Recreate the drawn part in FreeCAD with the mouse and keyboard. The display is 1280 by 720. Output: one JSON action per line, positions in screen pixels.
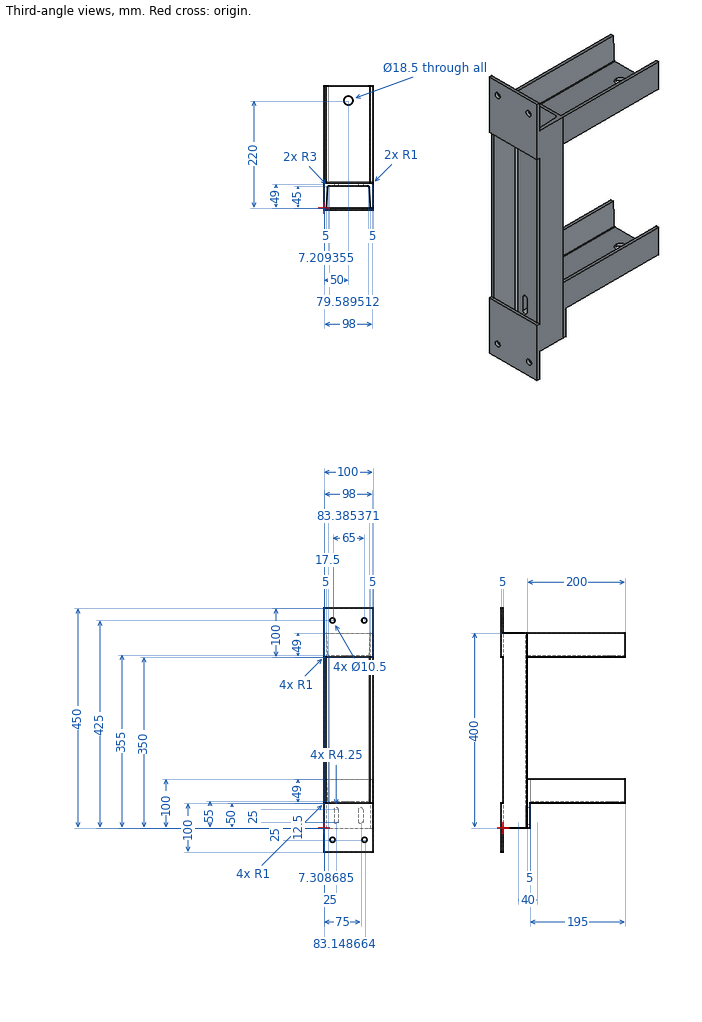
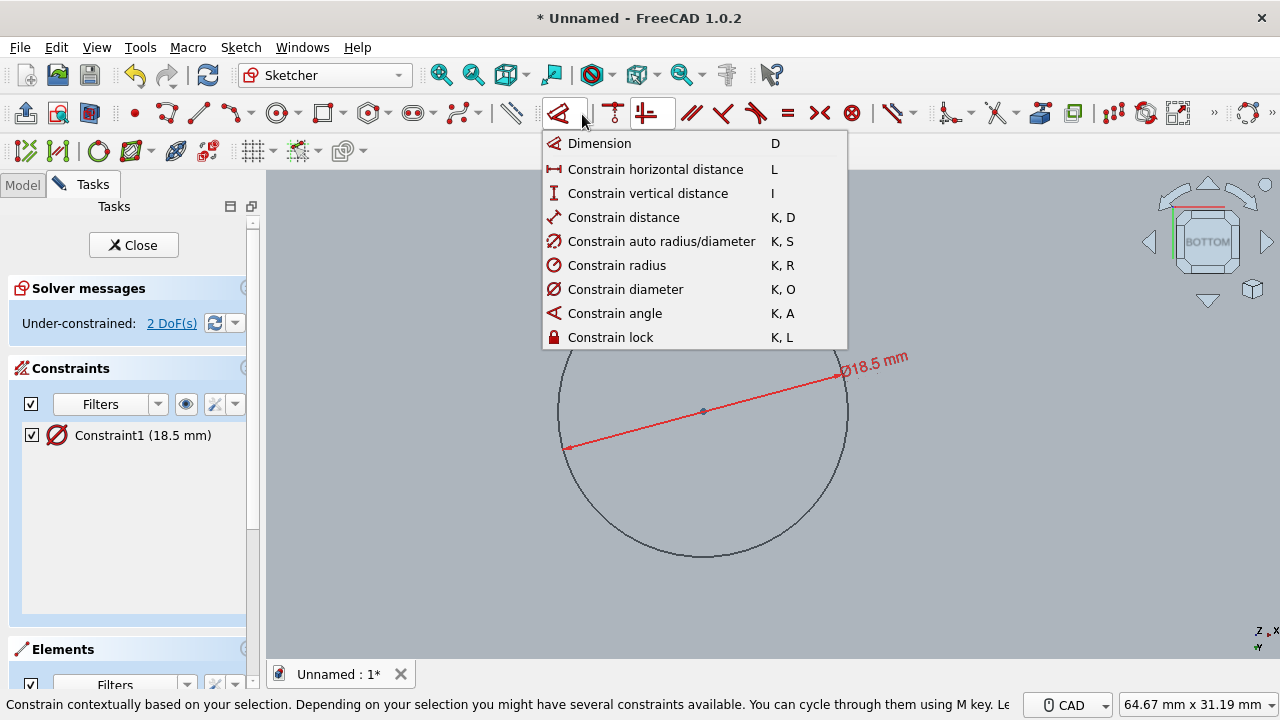
{"action": "left_click", "coordinate": [695, 169]}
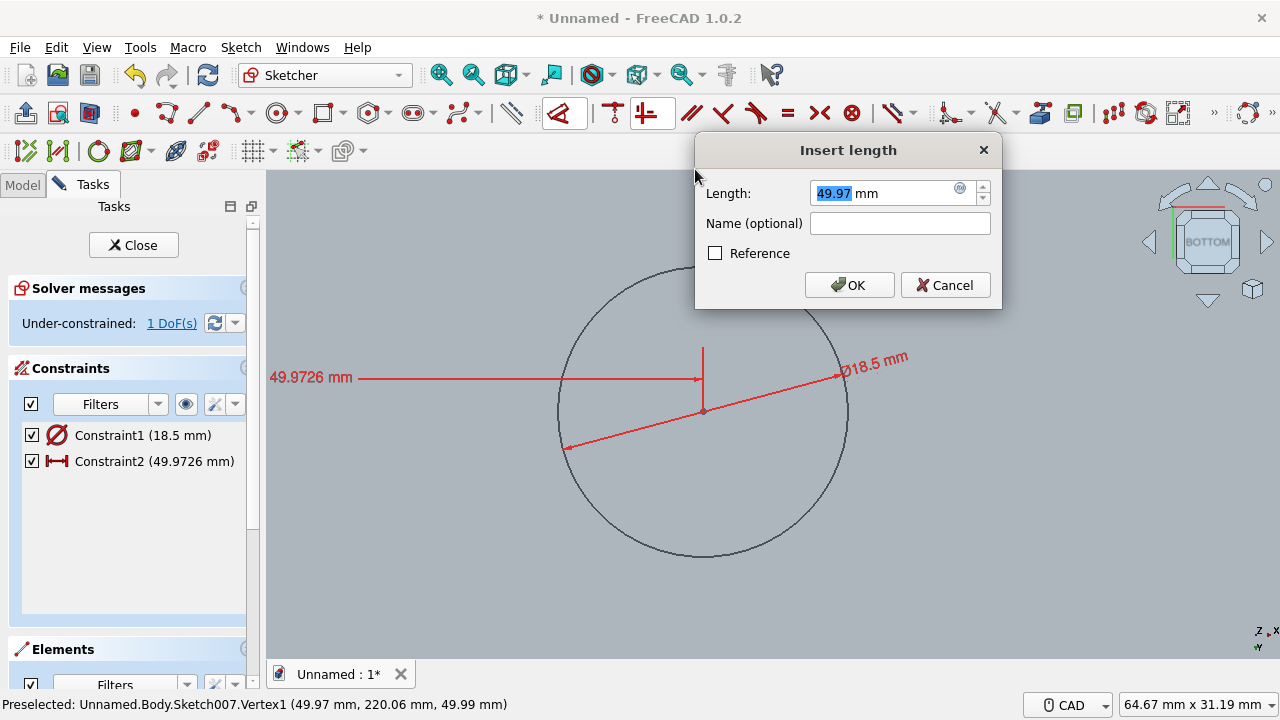
{"action": "type", "text": "50"}
{"action": "key", "text": "Return"}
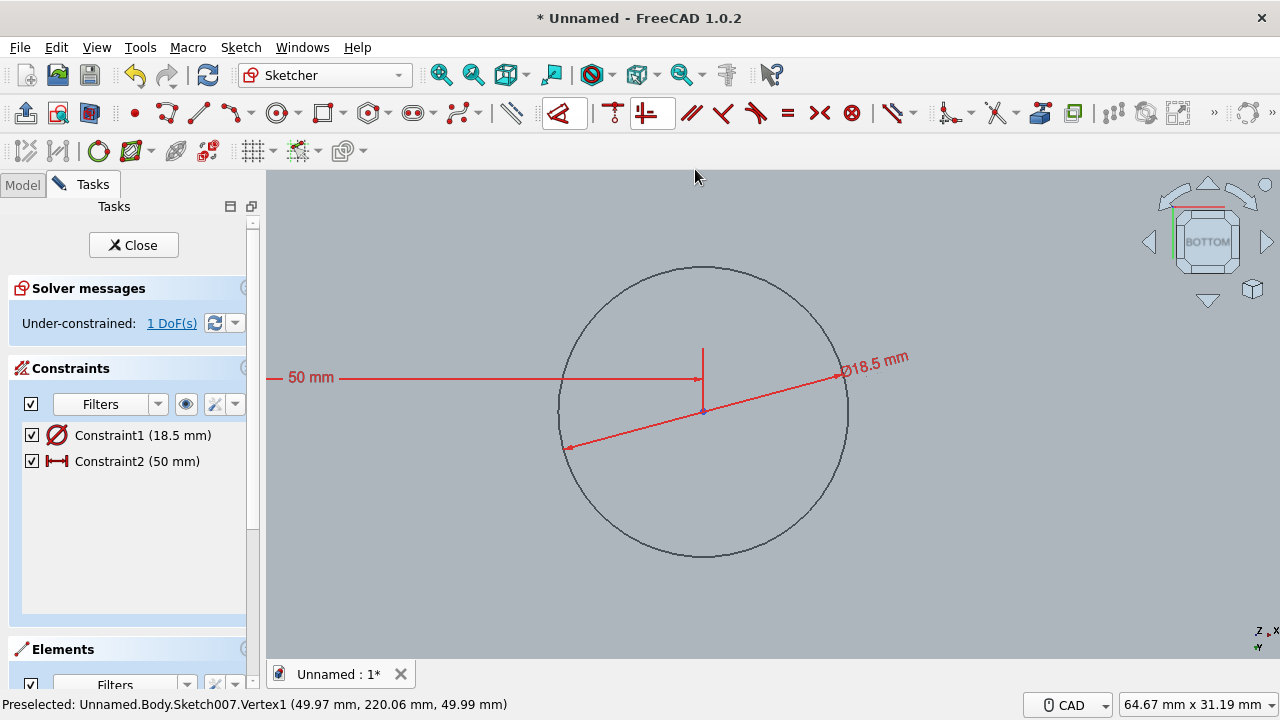
{"action": "left_click", "coordinate": [703, 412]}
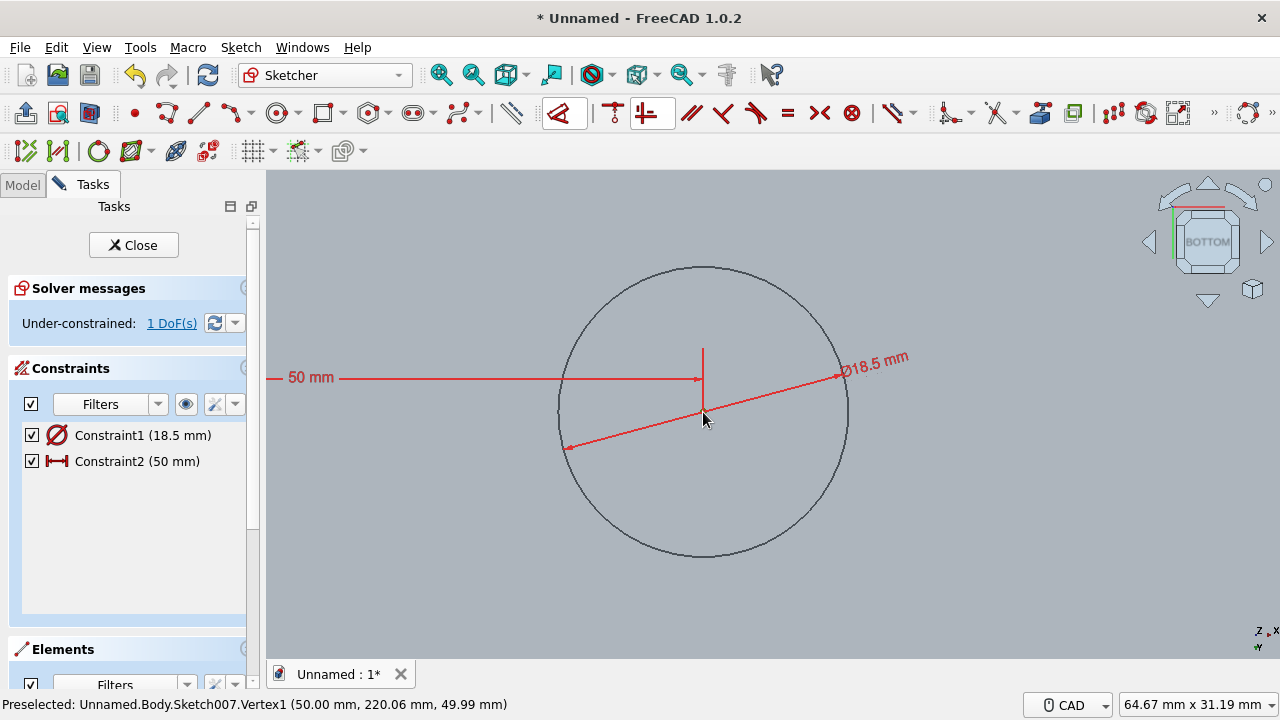
{"action": "left_click", "coordinate": [582, 114]}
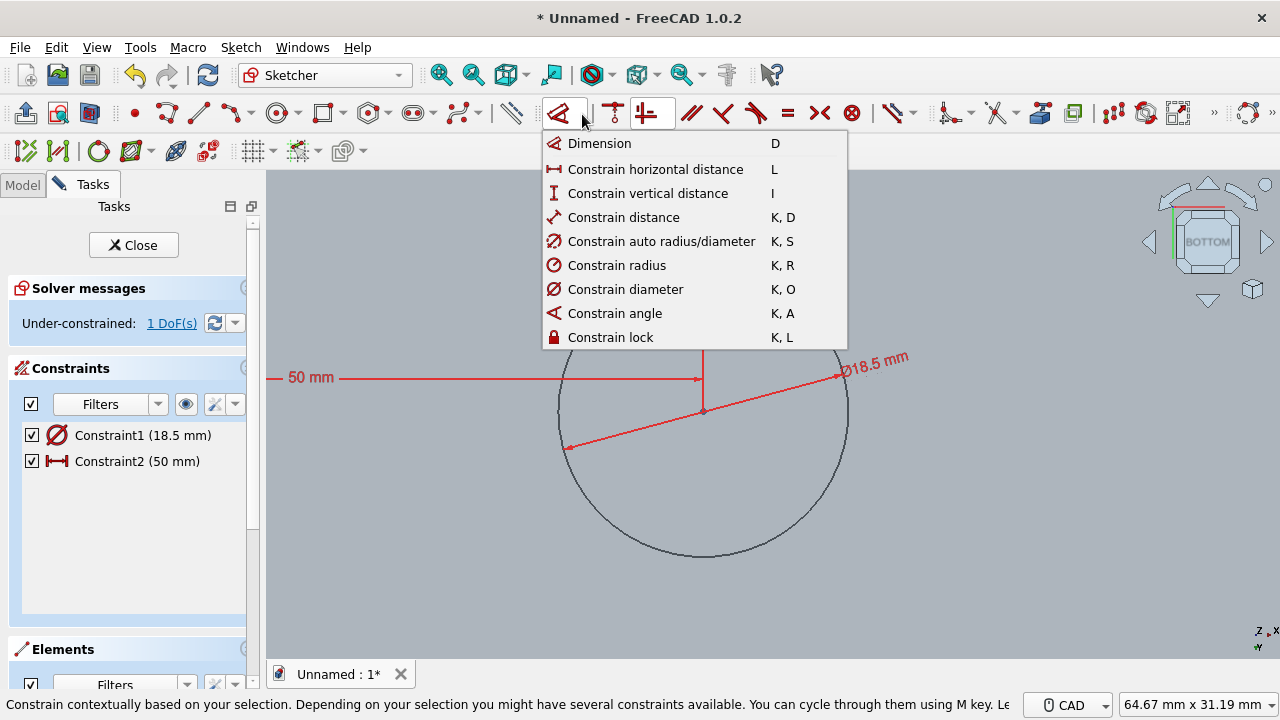
{"action": "left_click", "coordinate": [695, 193]}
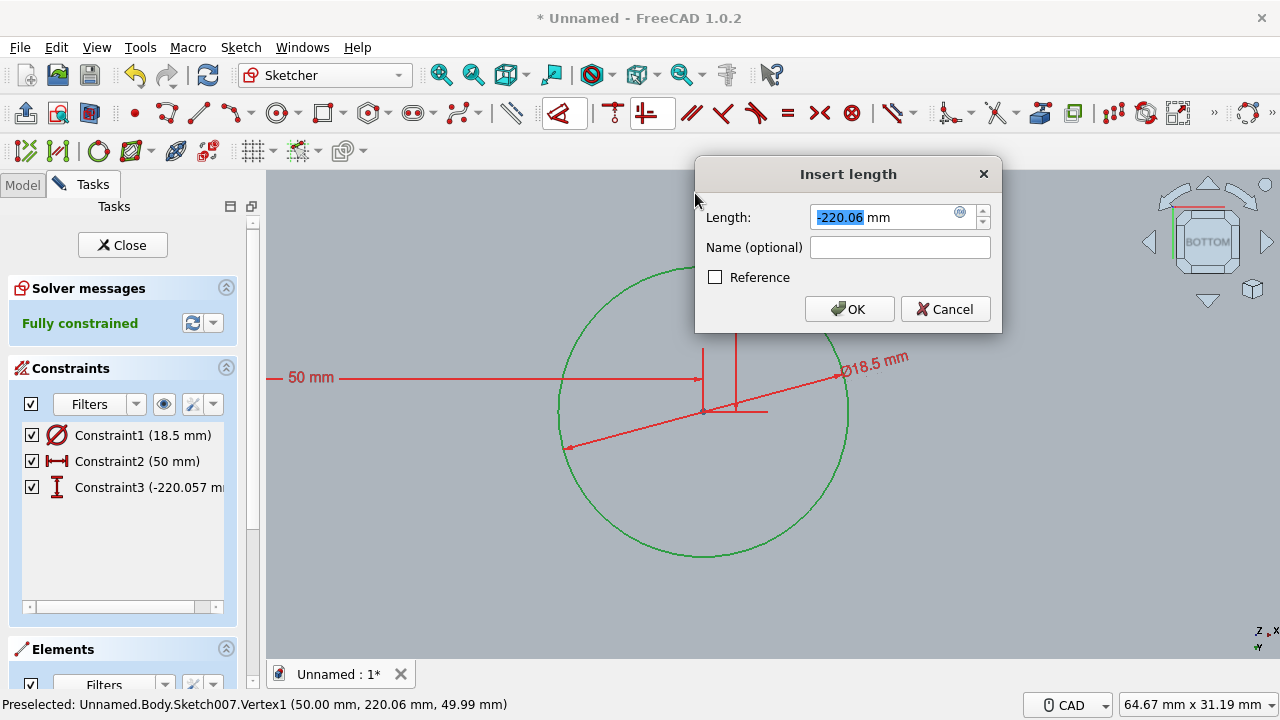
{"action": "type", "text": "-220"}
{"action": "key", "text": "Return"}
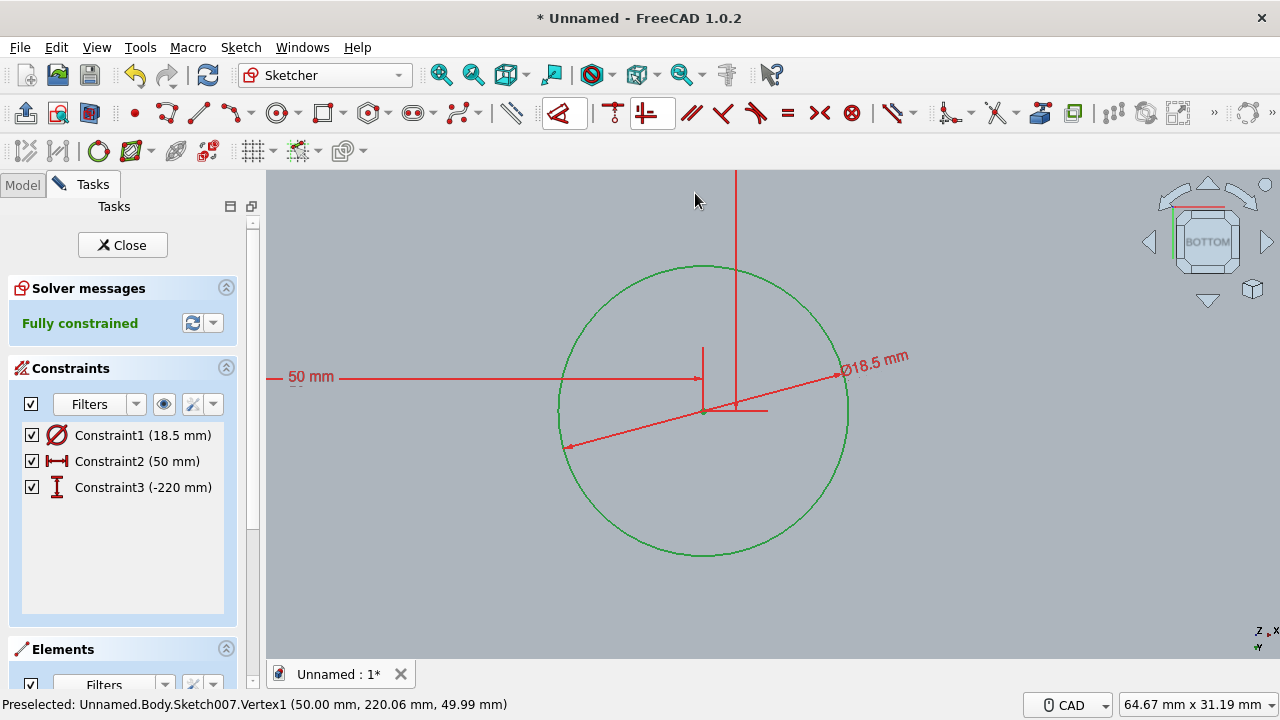
{"action": "left_click", "coordinate": [123, 245]}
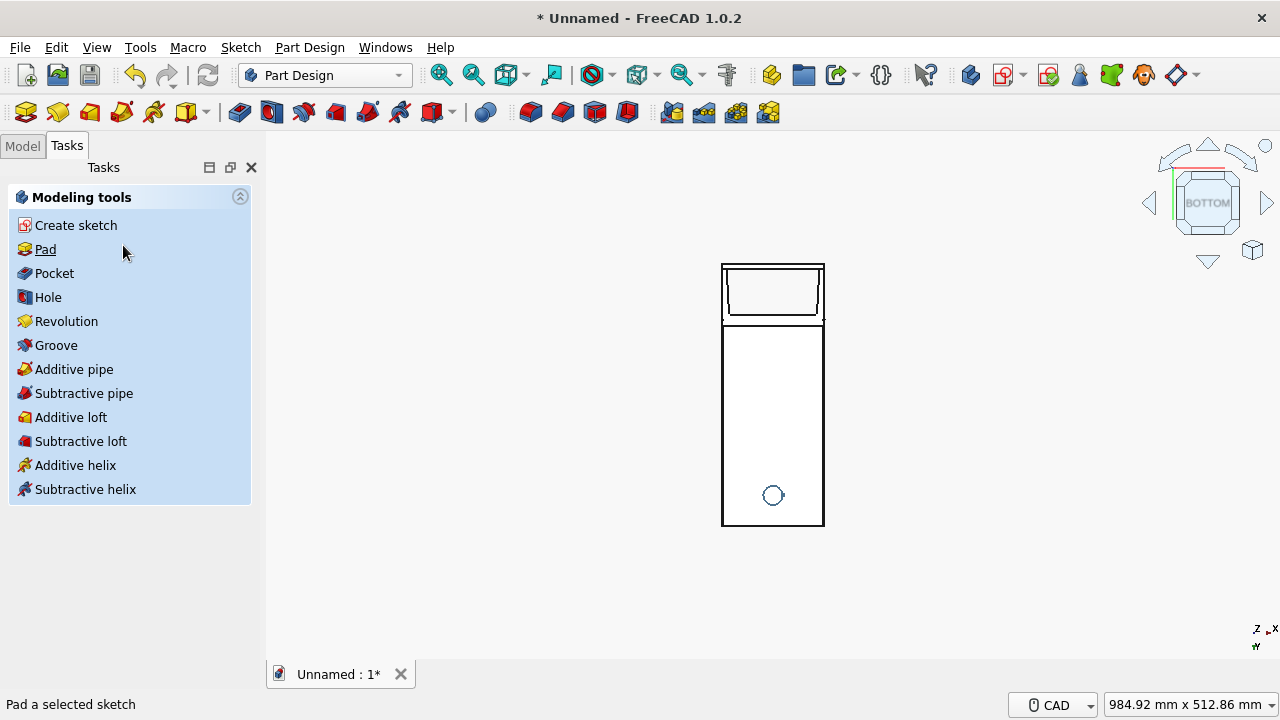
{"action": "left_click", "coordinate": [272, 112]}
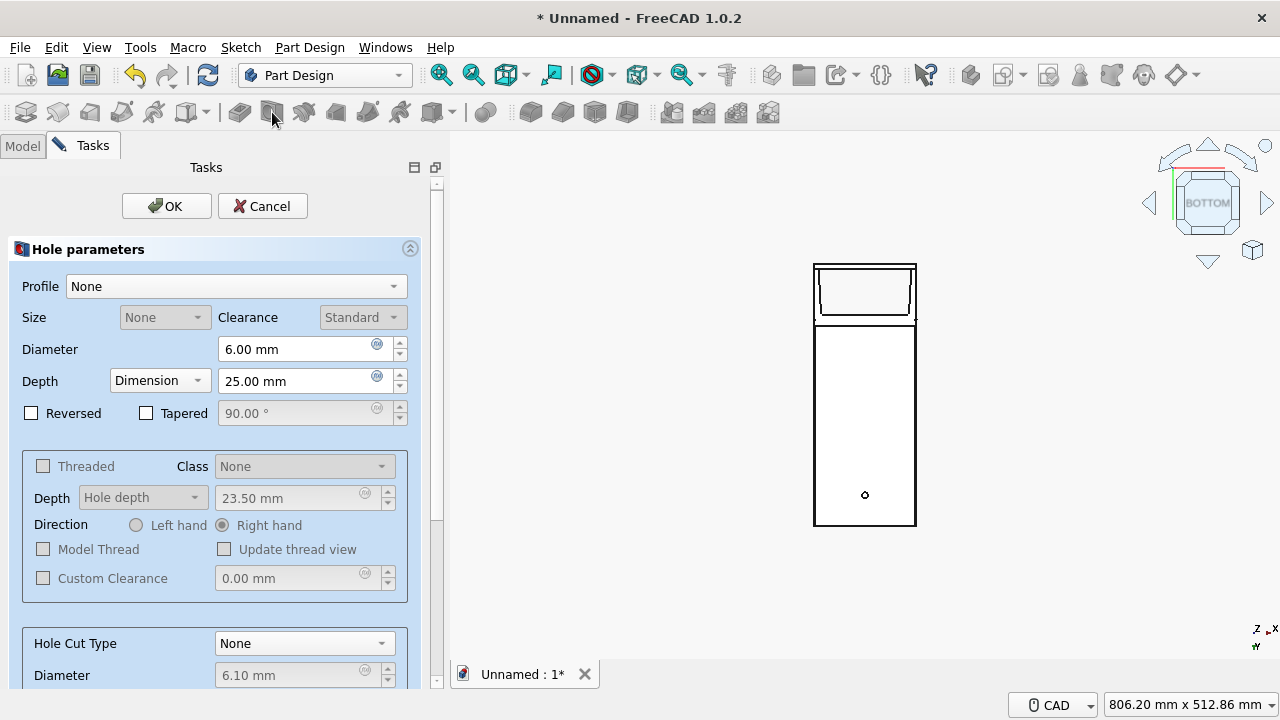
{"action": "triple_click", "coordinate": [305, 349]}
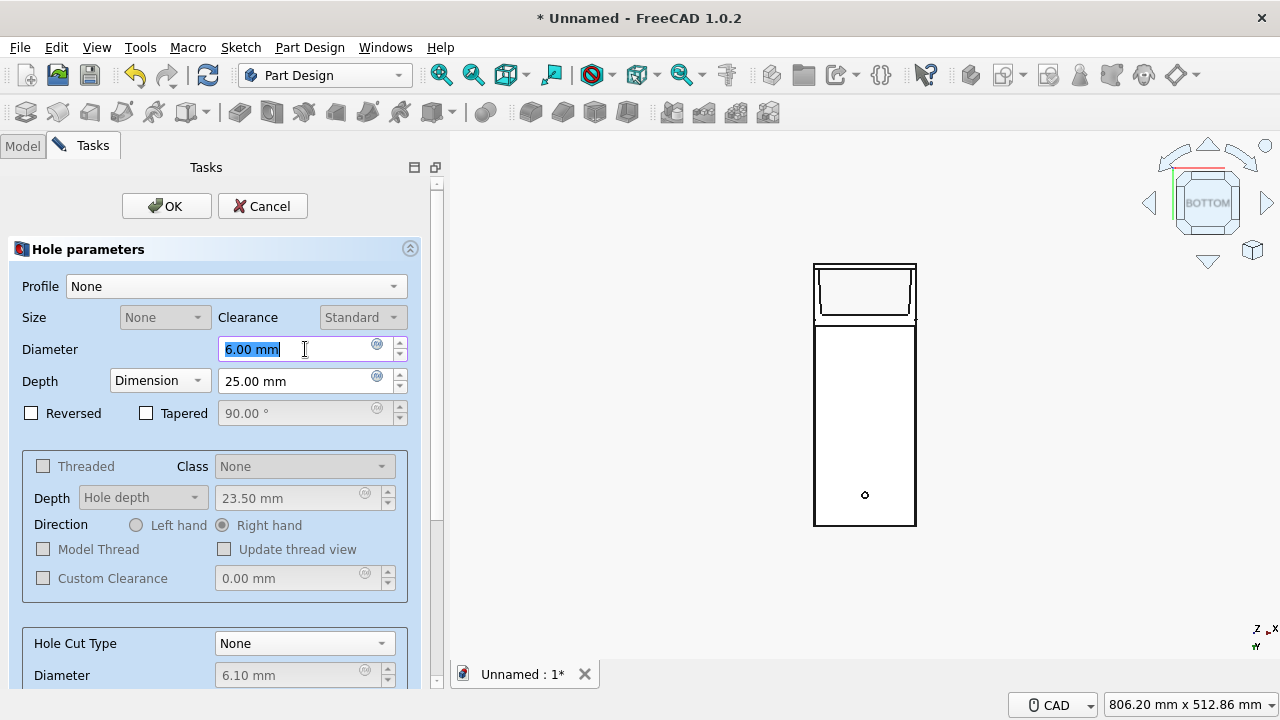
{"action": "type", "text": "18.5"}
{"action": "key", "text": "Tab"}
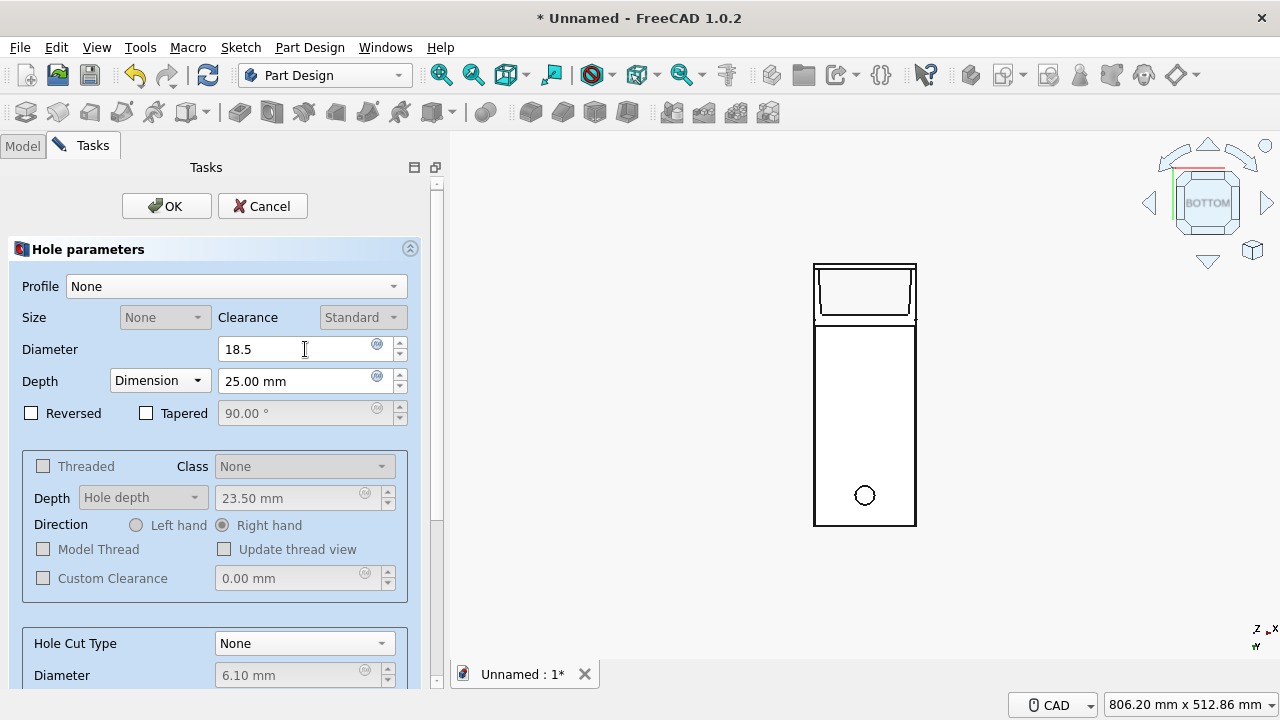
{"action": "left_click", "coordinate": [161, 380]}